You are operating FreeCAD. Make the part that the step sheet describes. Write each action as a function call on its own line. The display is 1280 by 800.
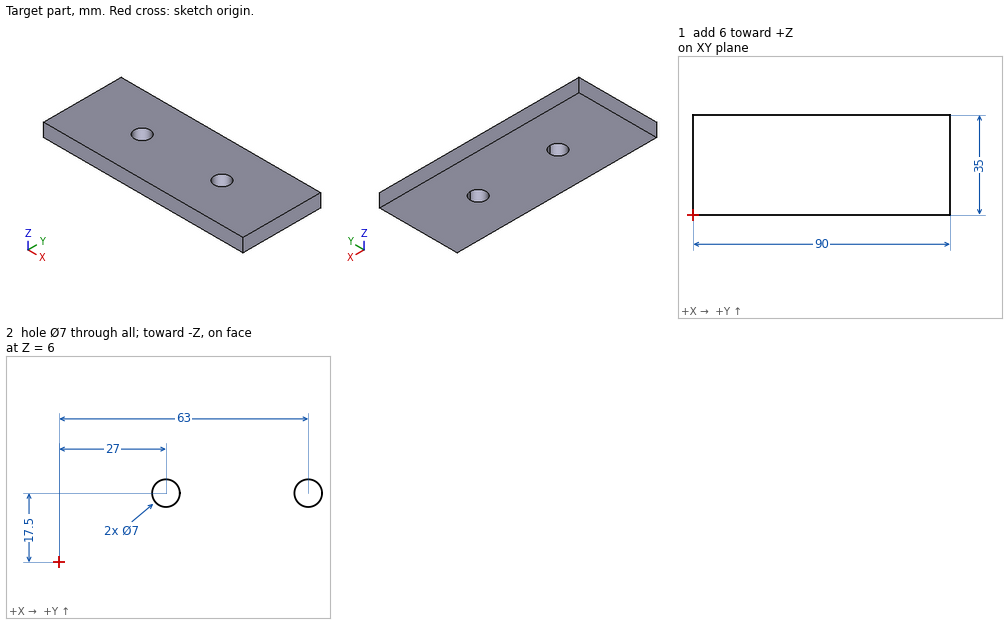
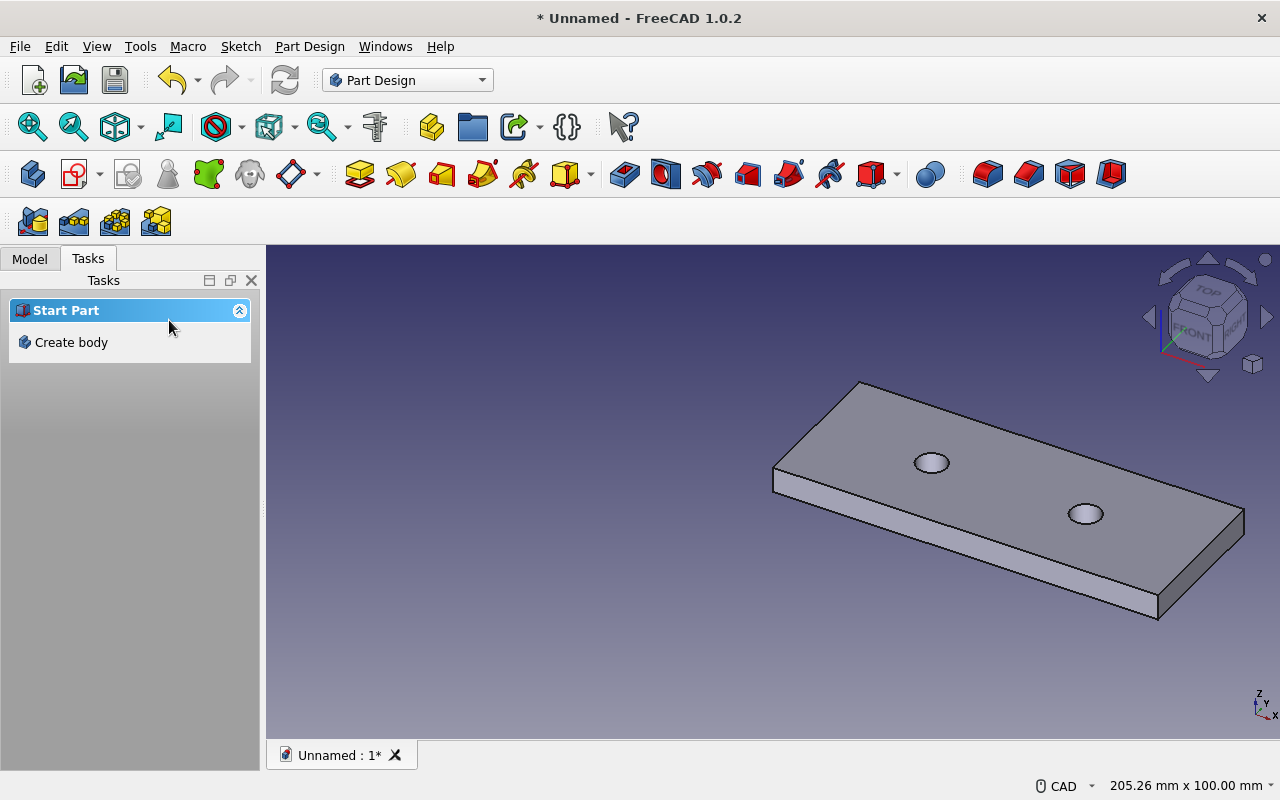
key(0)